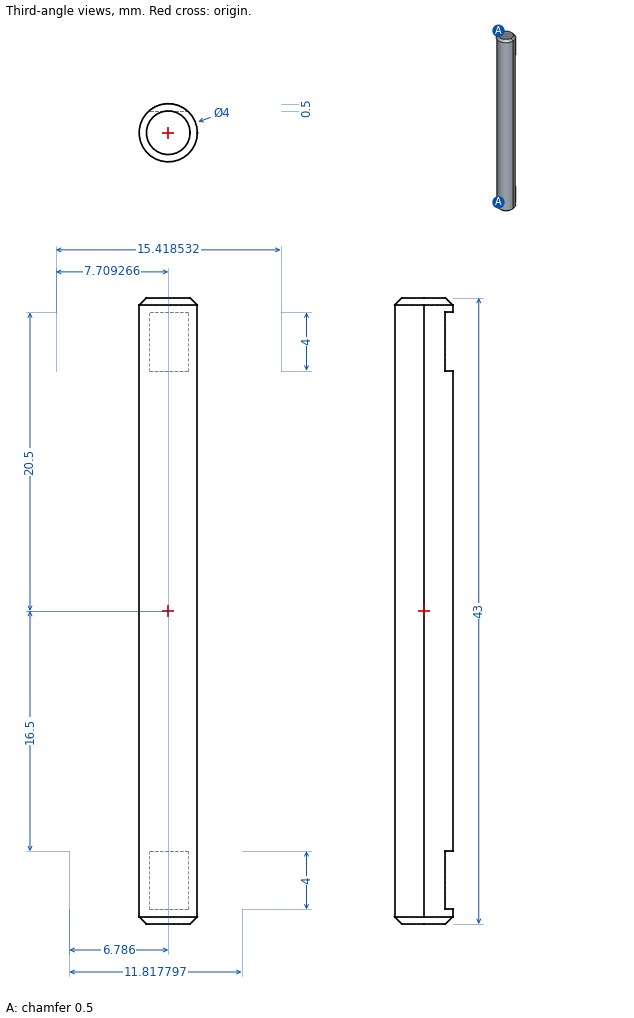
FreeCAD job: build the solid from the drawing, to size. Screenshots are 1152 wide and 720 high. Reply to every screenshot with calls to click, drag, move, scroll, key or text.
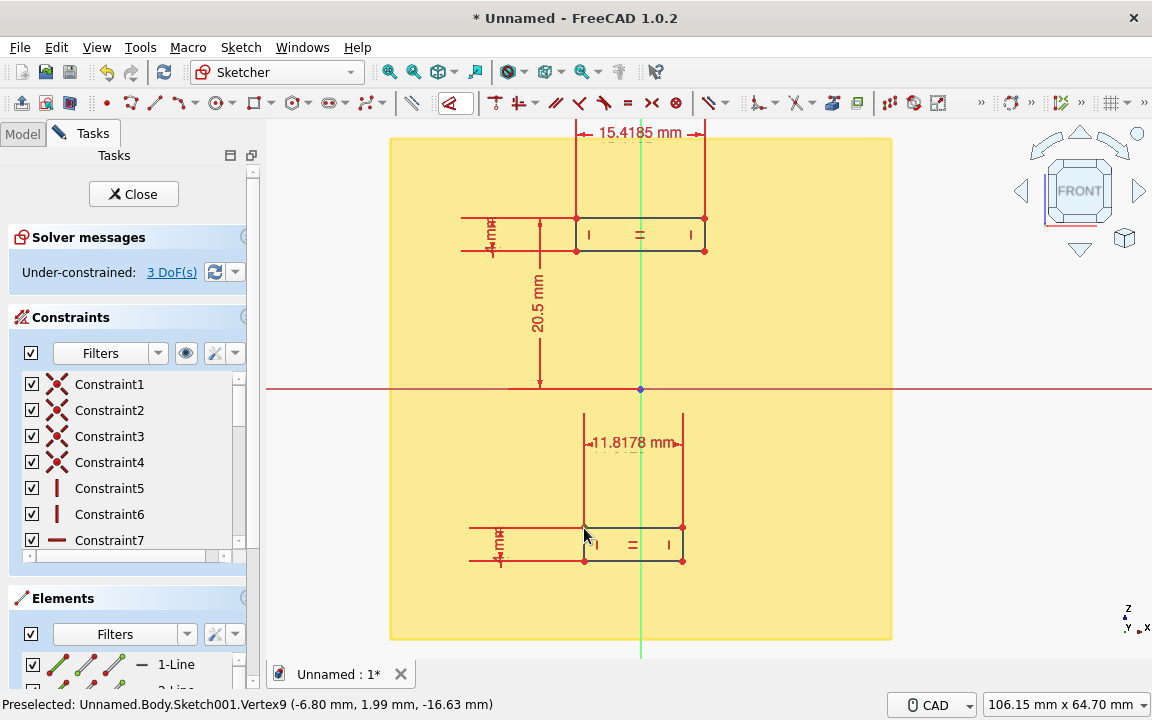
key(i)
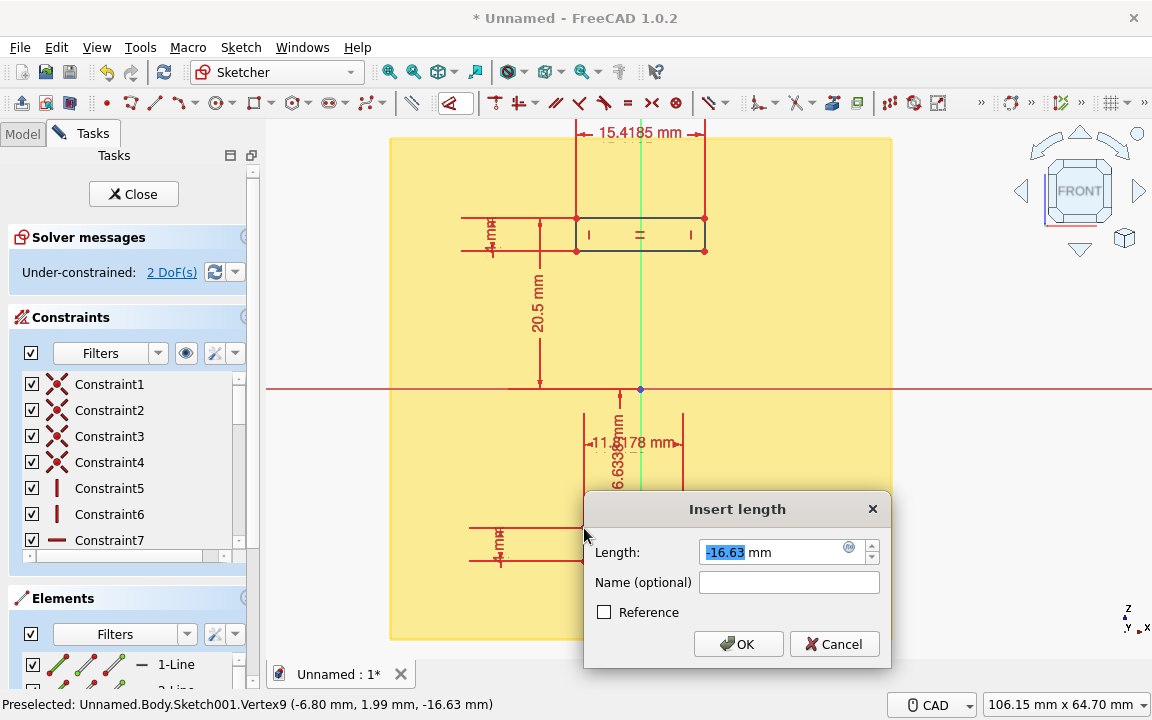
text(-16.5)
key(Return)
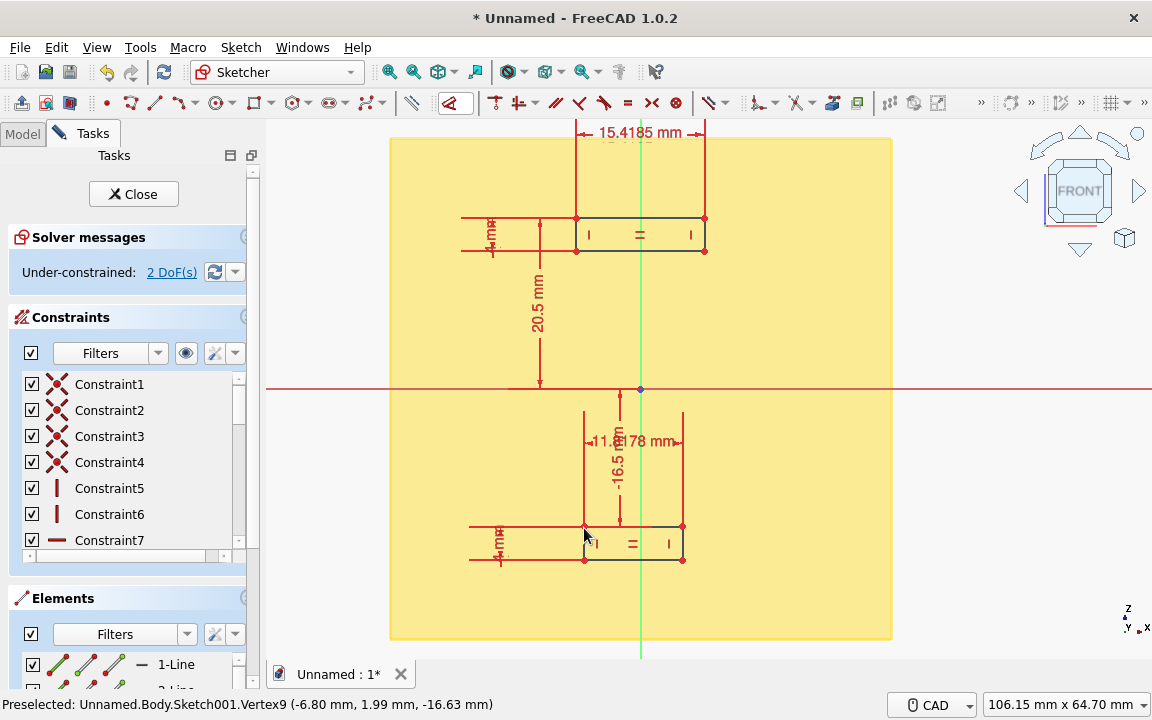
click(584, 527)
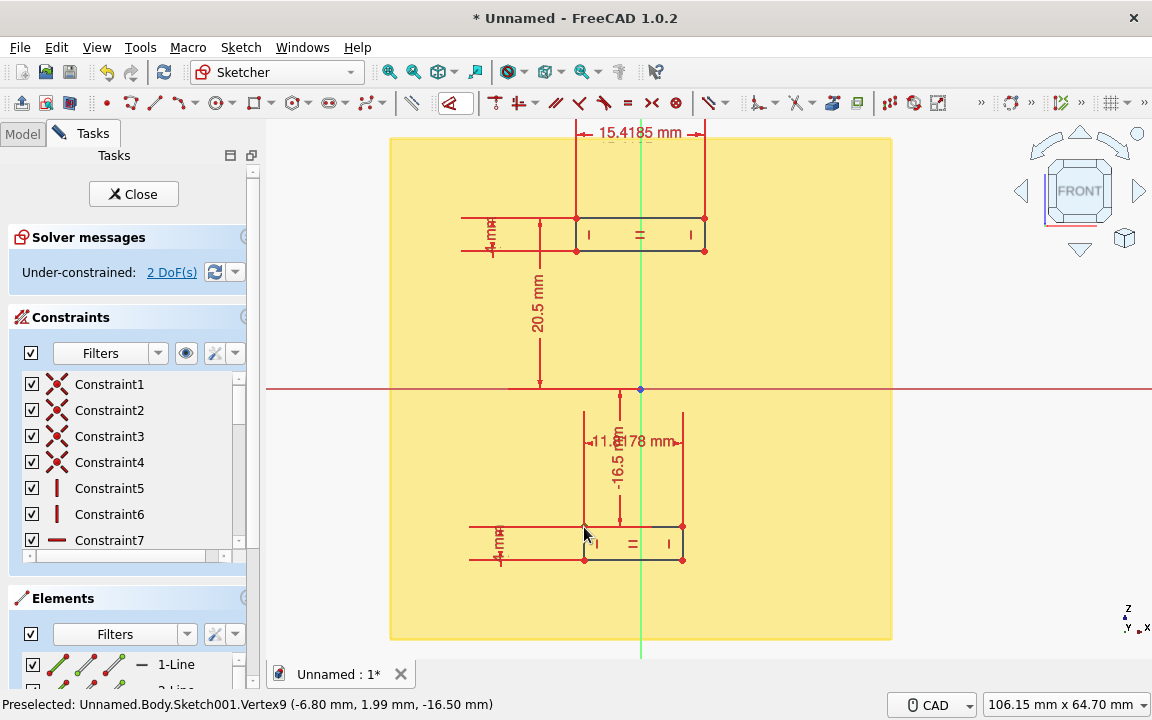
key(l)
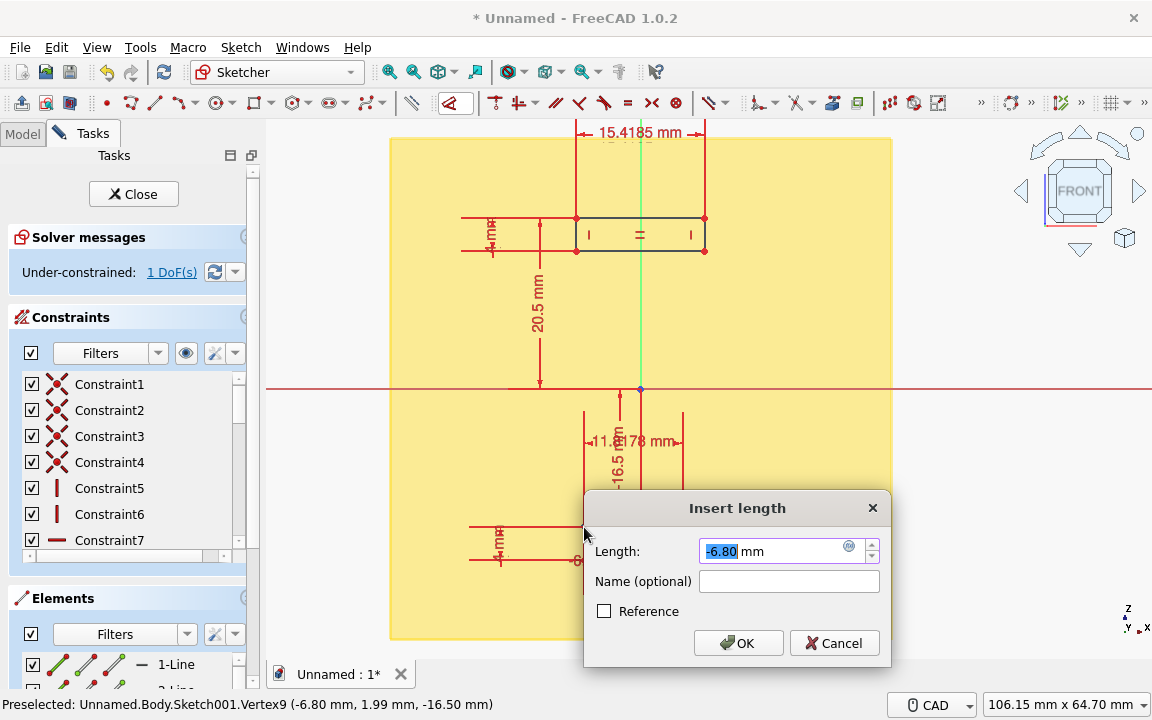
text(-6.786)
key(Return)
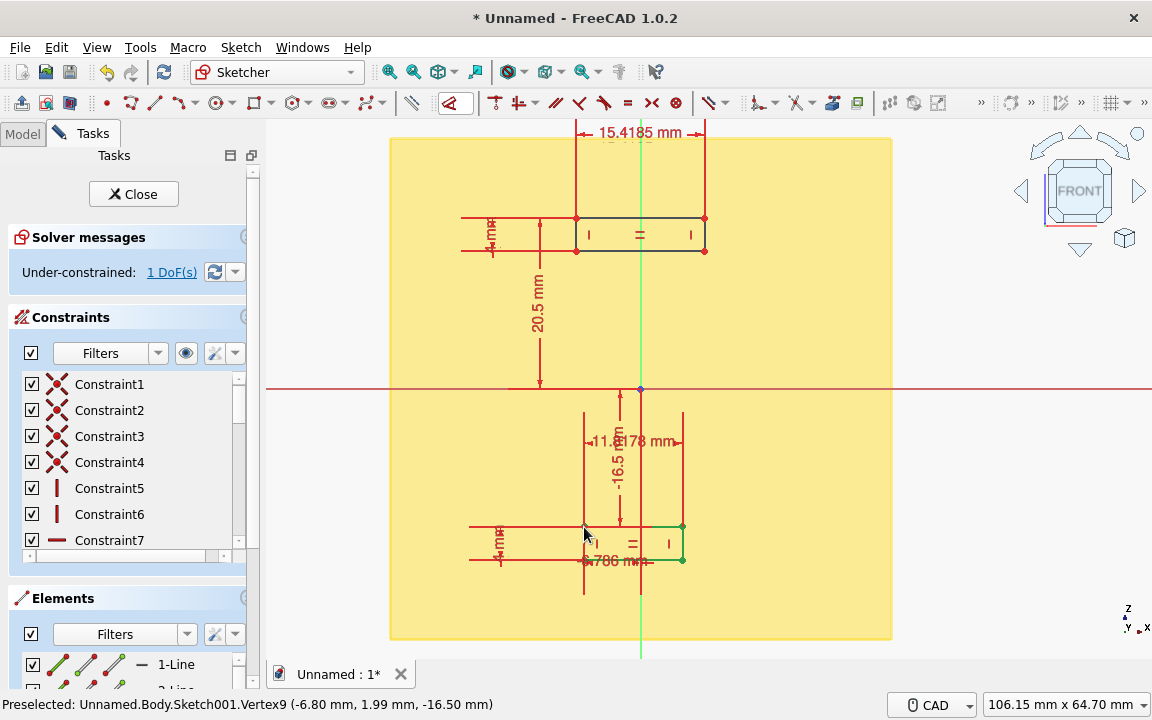
click(576, 218)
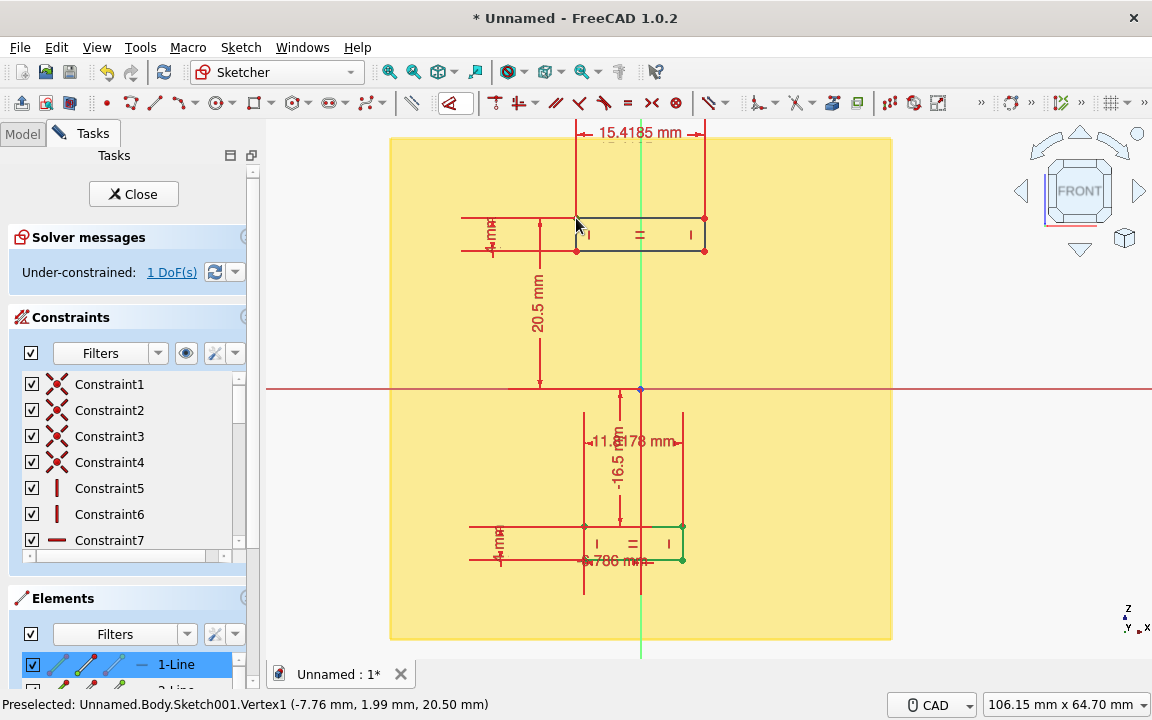
click(468, 104)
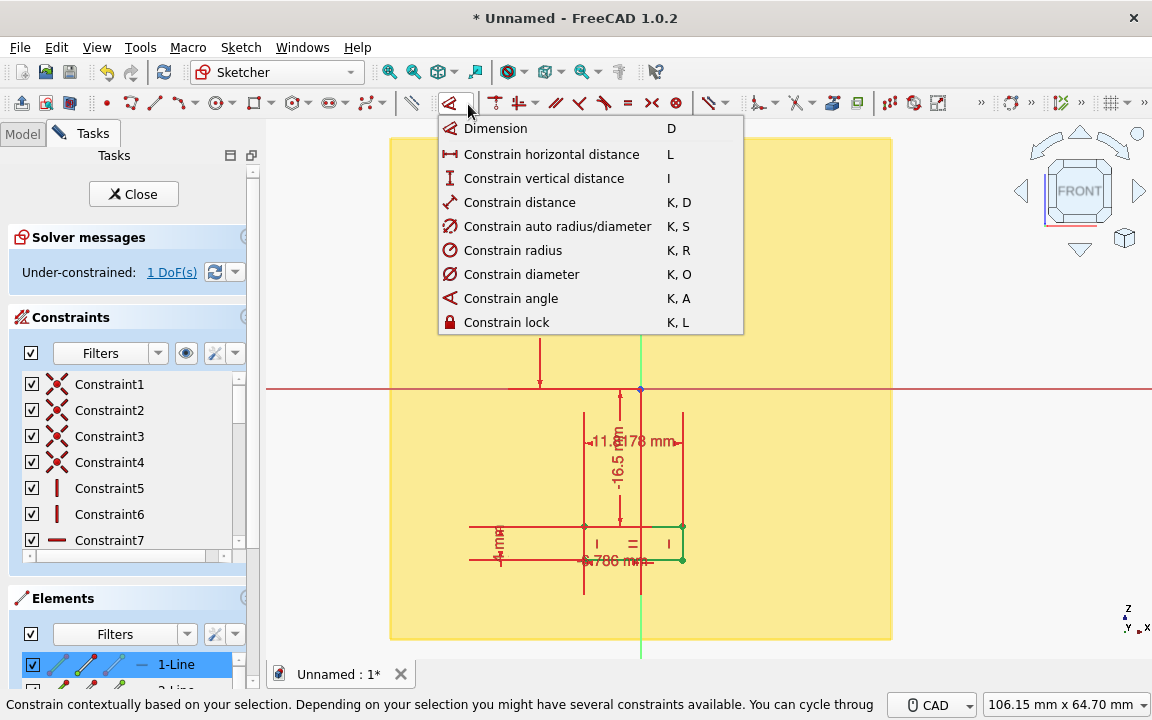
click(591, 154)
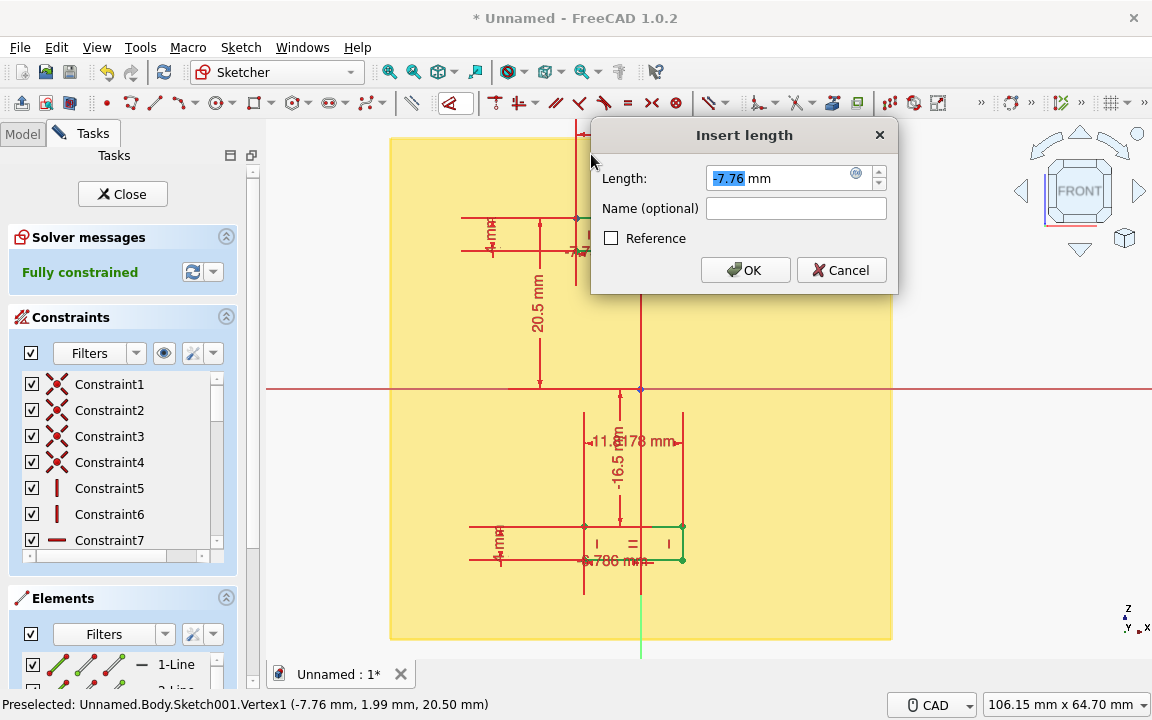
text(-7.709266)
key(Return)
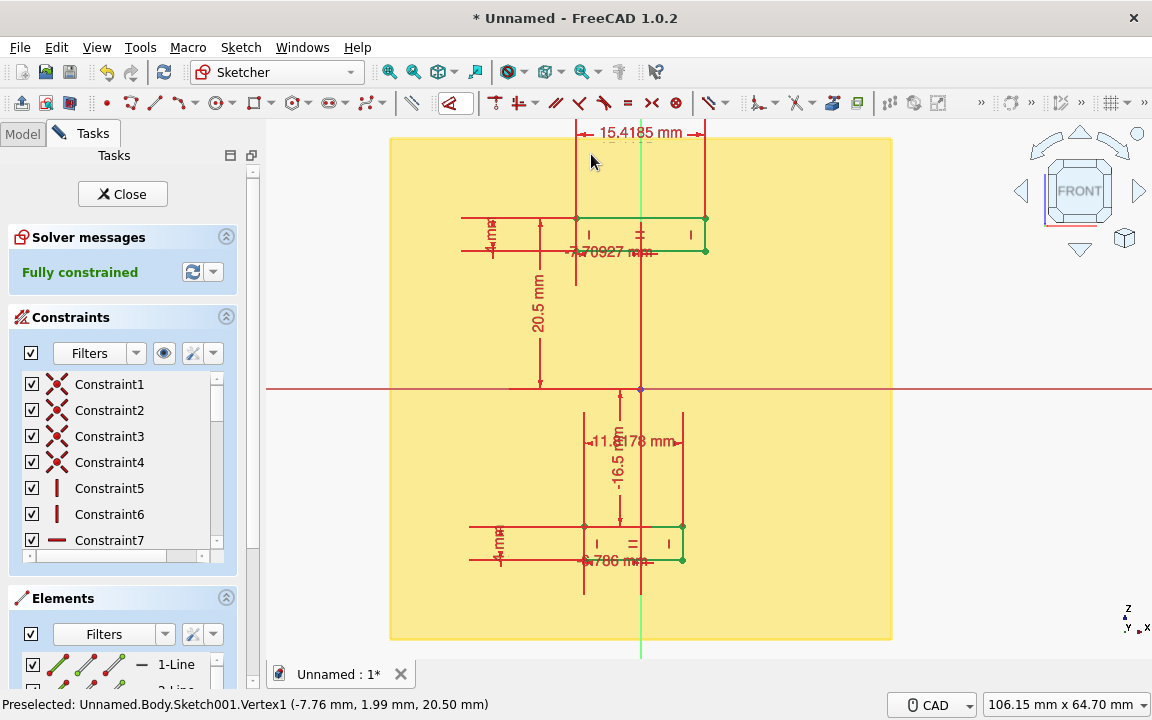
click(123, 194)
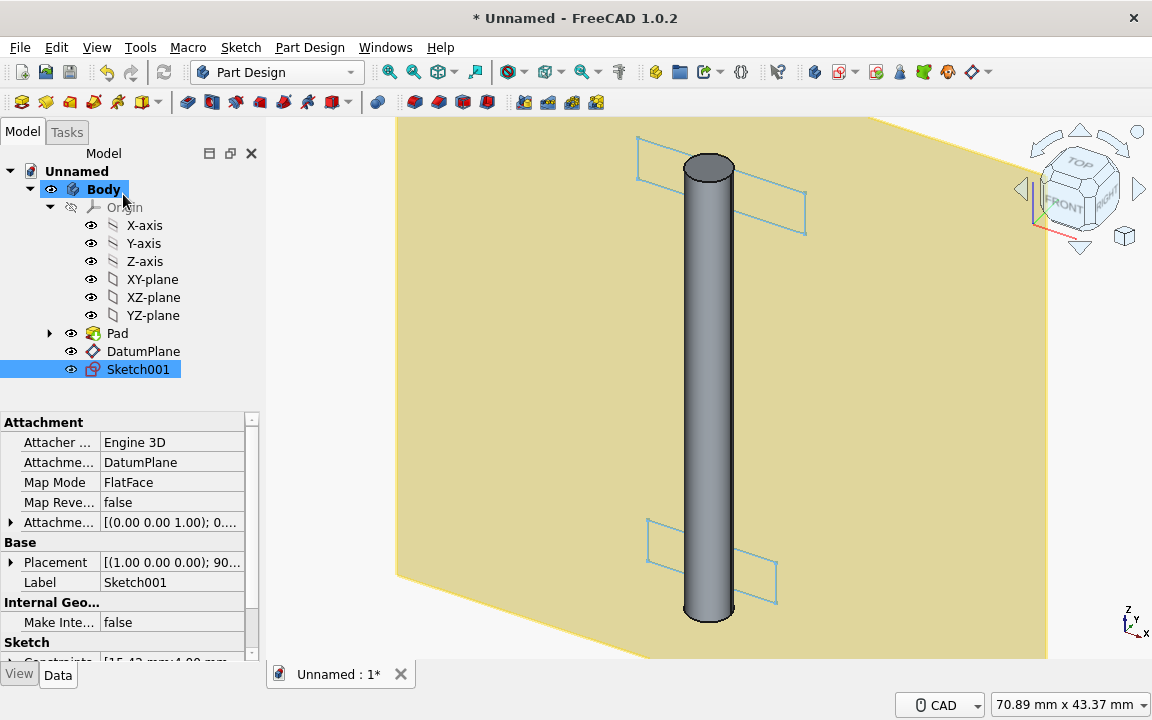
click(188, 102)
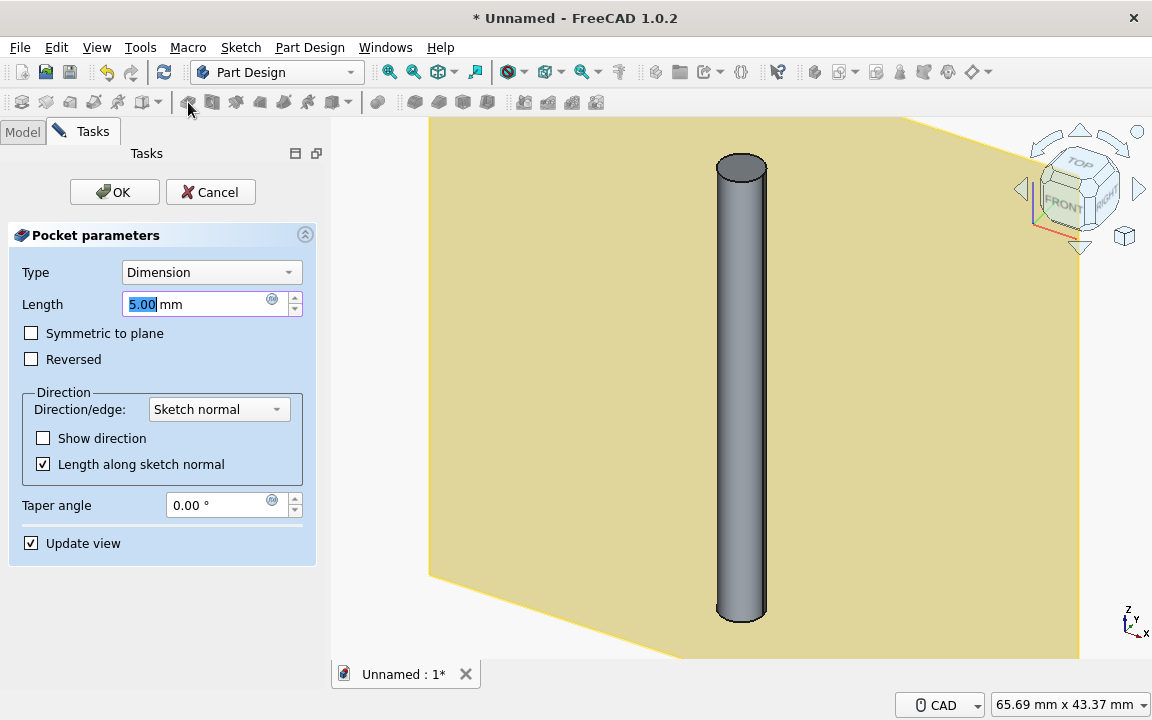
text(0.5)
key(Tab)